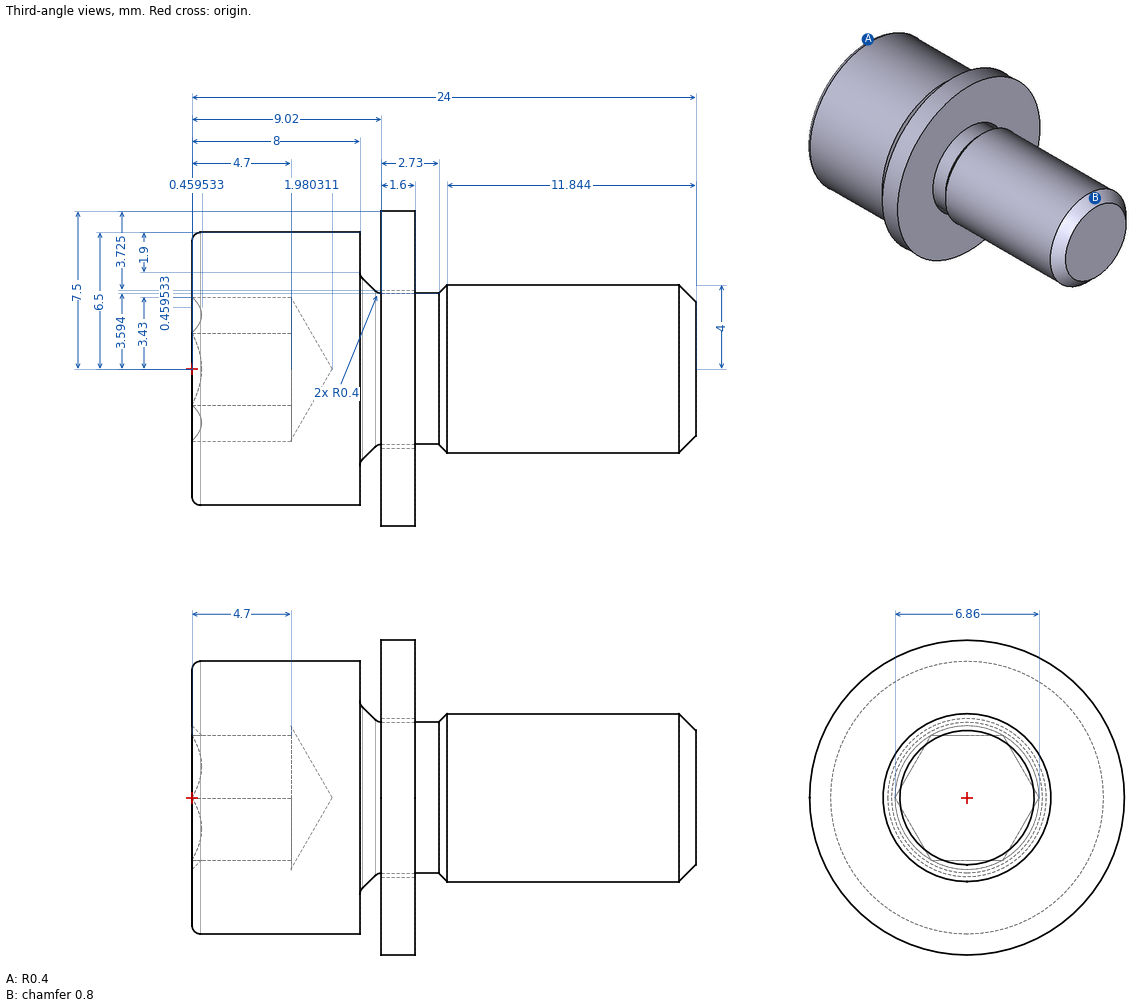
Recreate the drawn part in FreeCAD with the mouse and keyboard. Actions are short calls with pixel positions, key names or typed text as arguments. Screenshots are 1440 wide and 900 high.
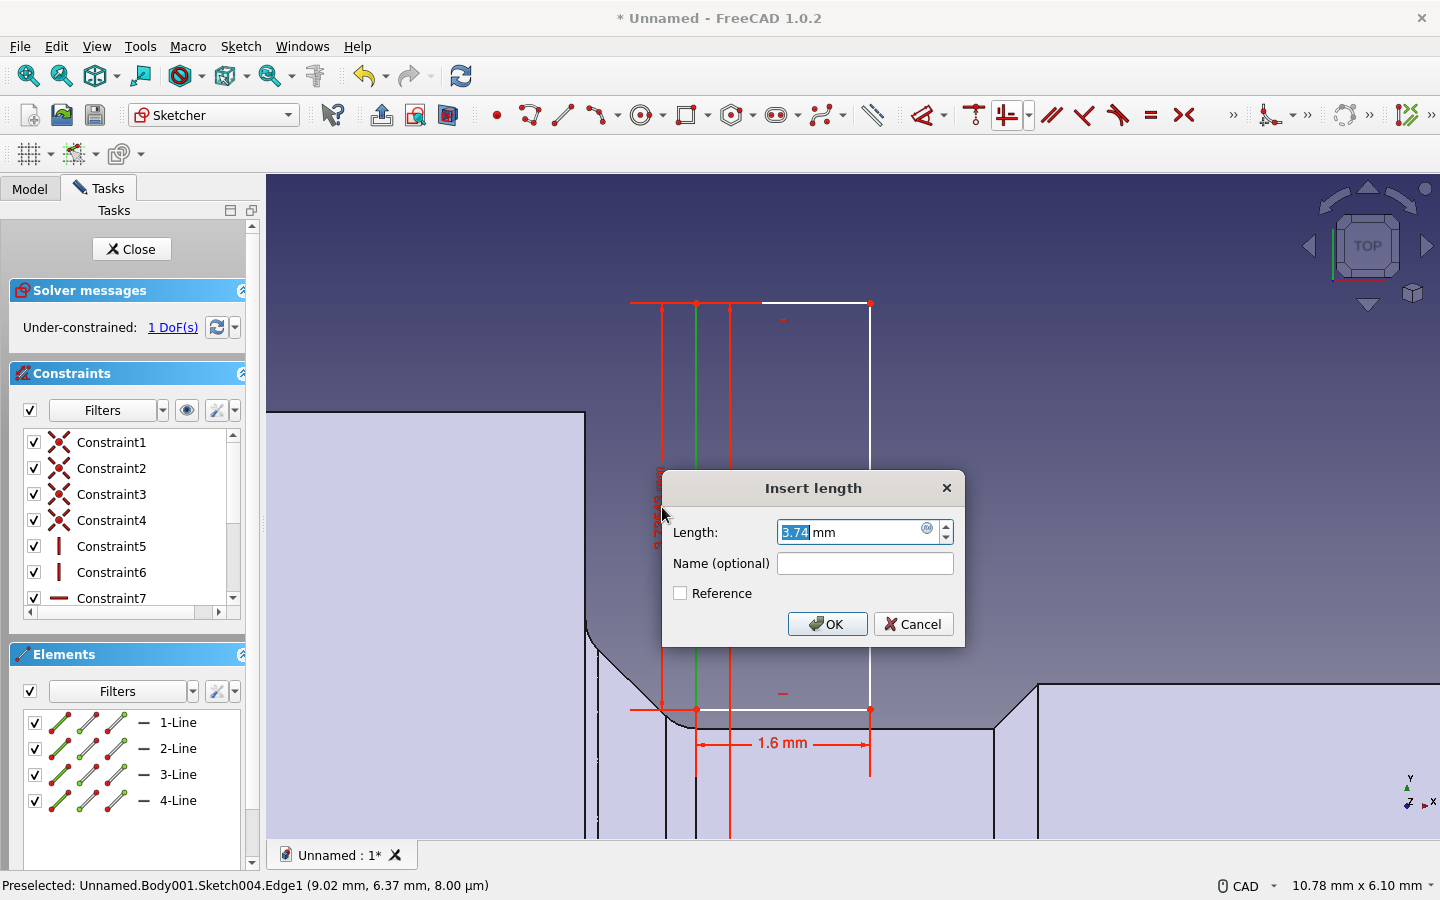
text(3.725)
key(Return)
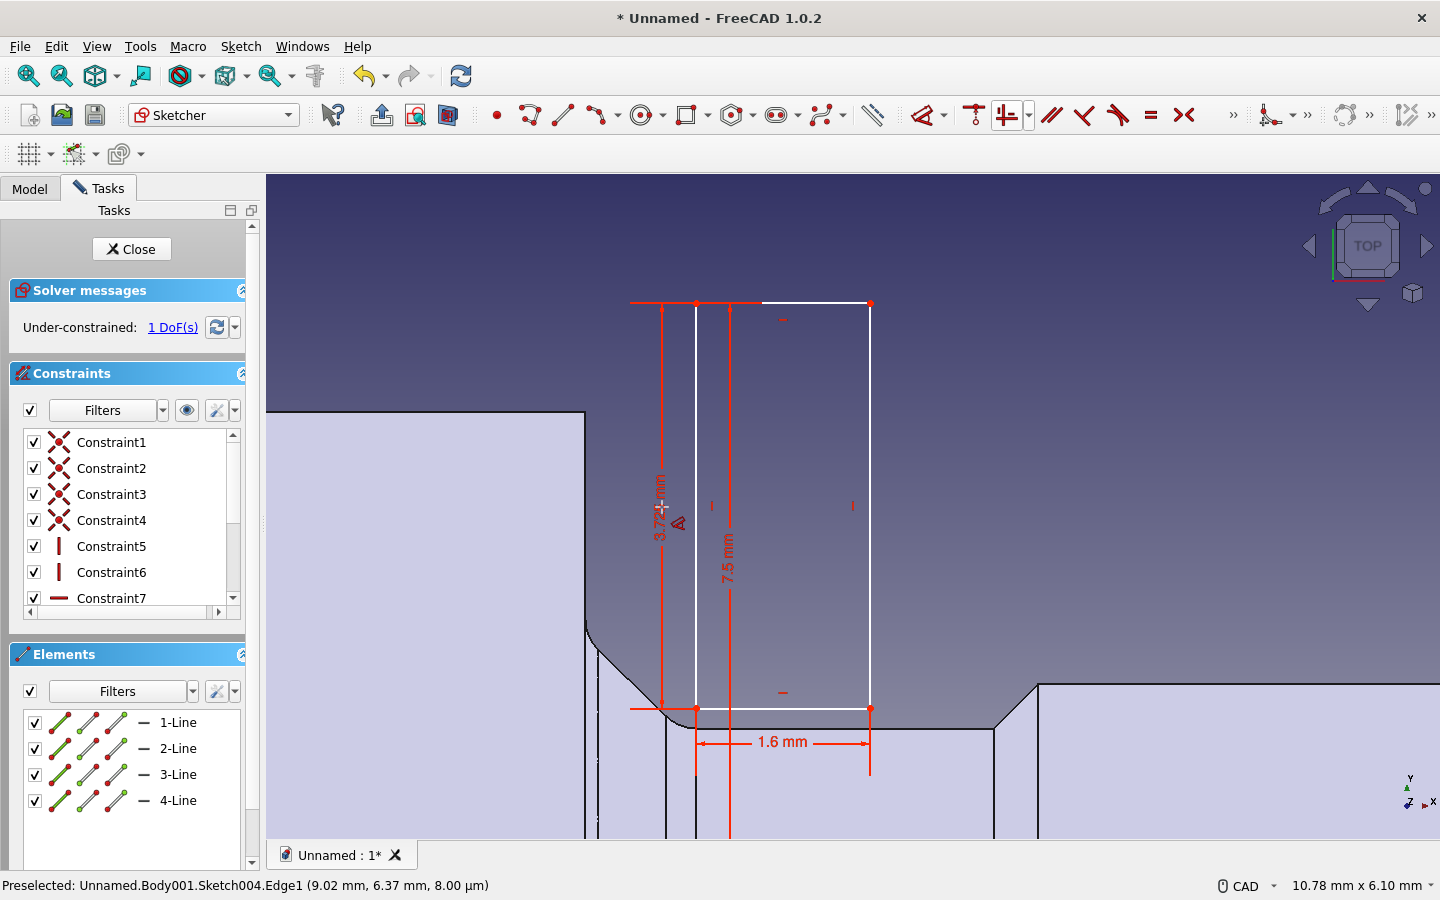
click(696, 303)
click(495, 269)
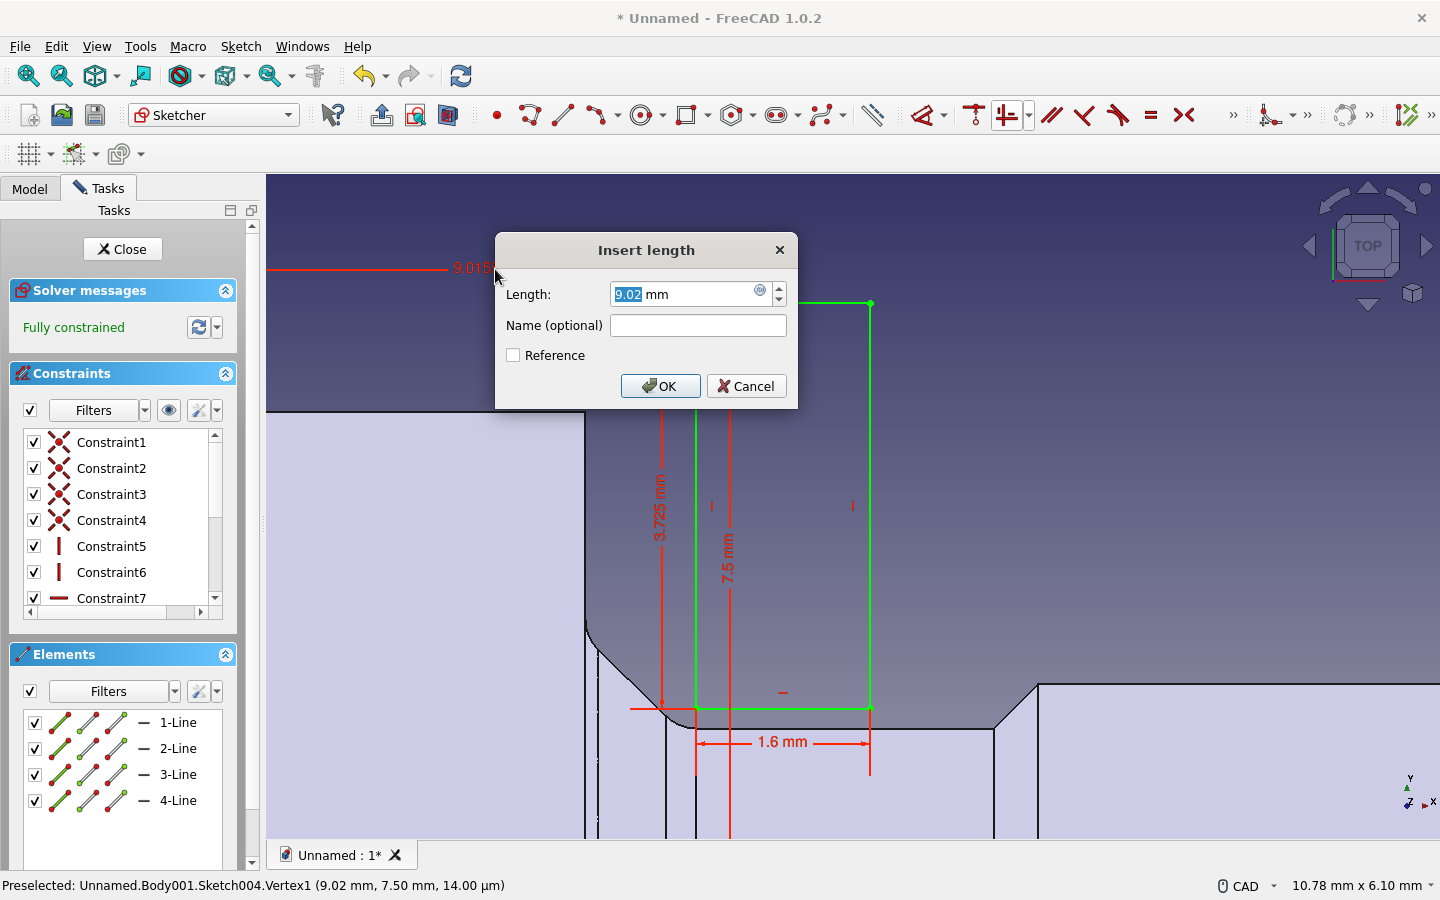
text(9.02)
key(Return)
key(Escape)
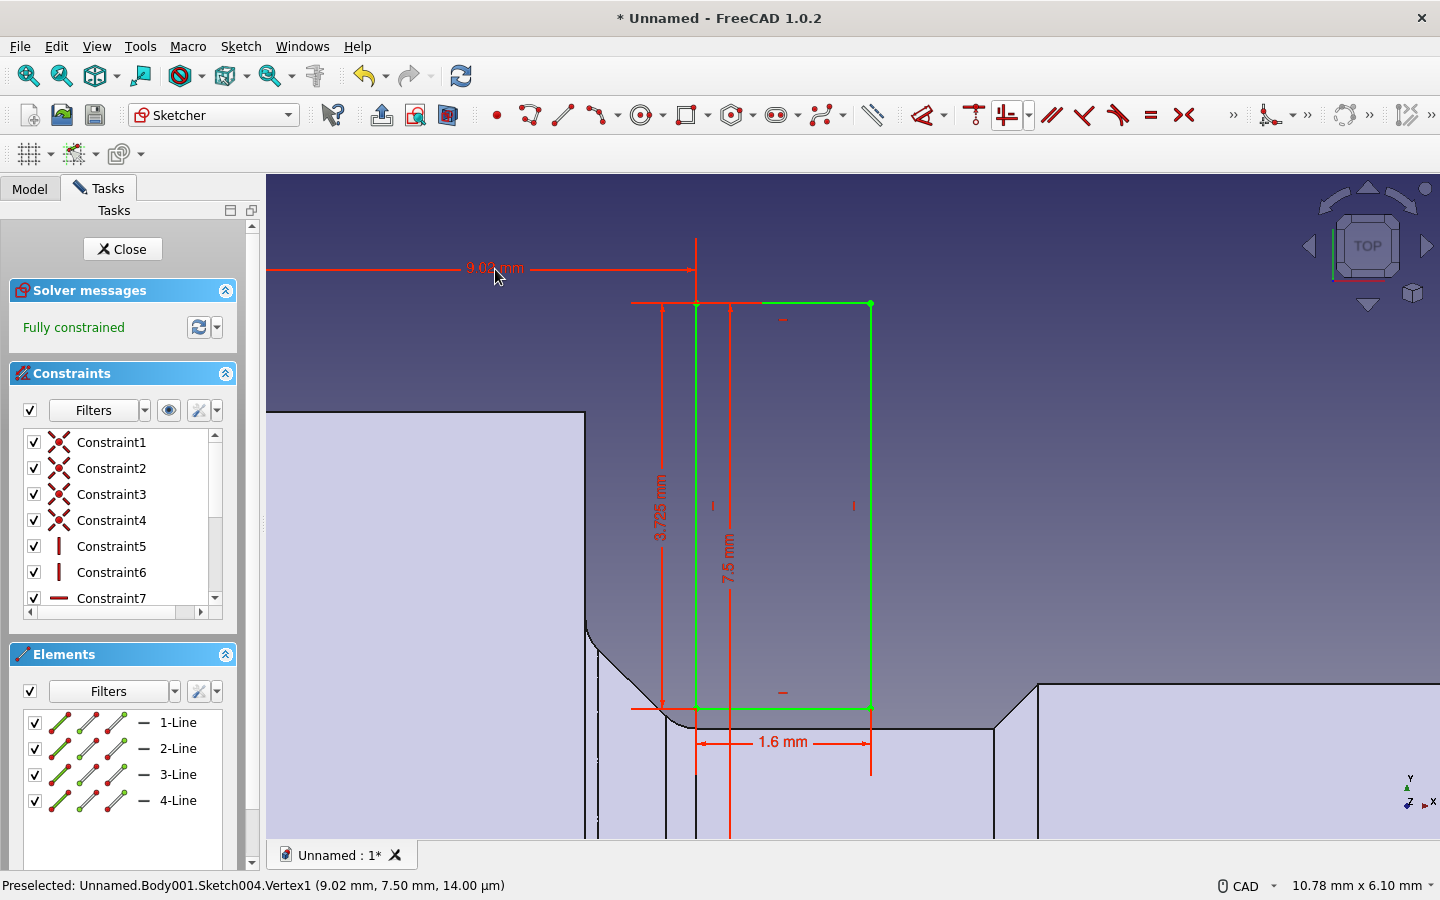
click(123, 249)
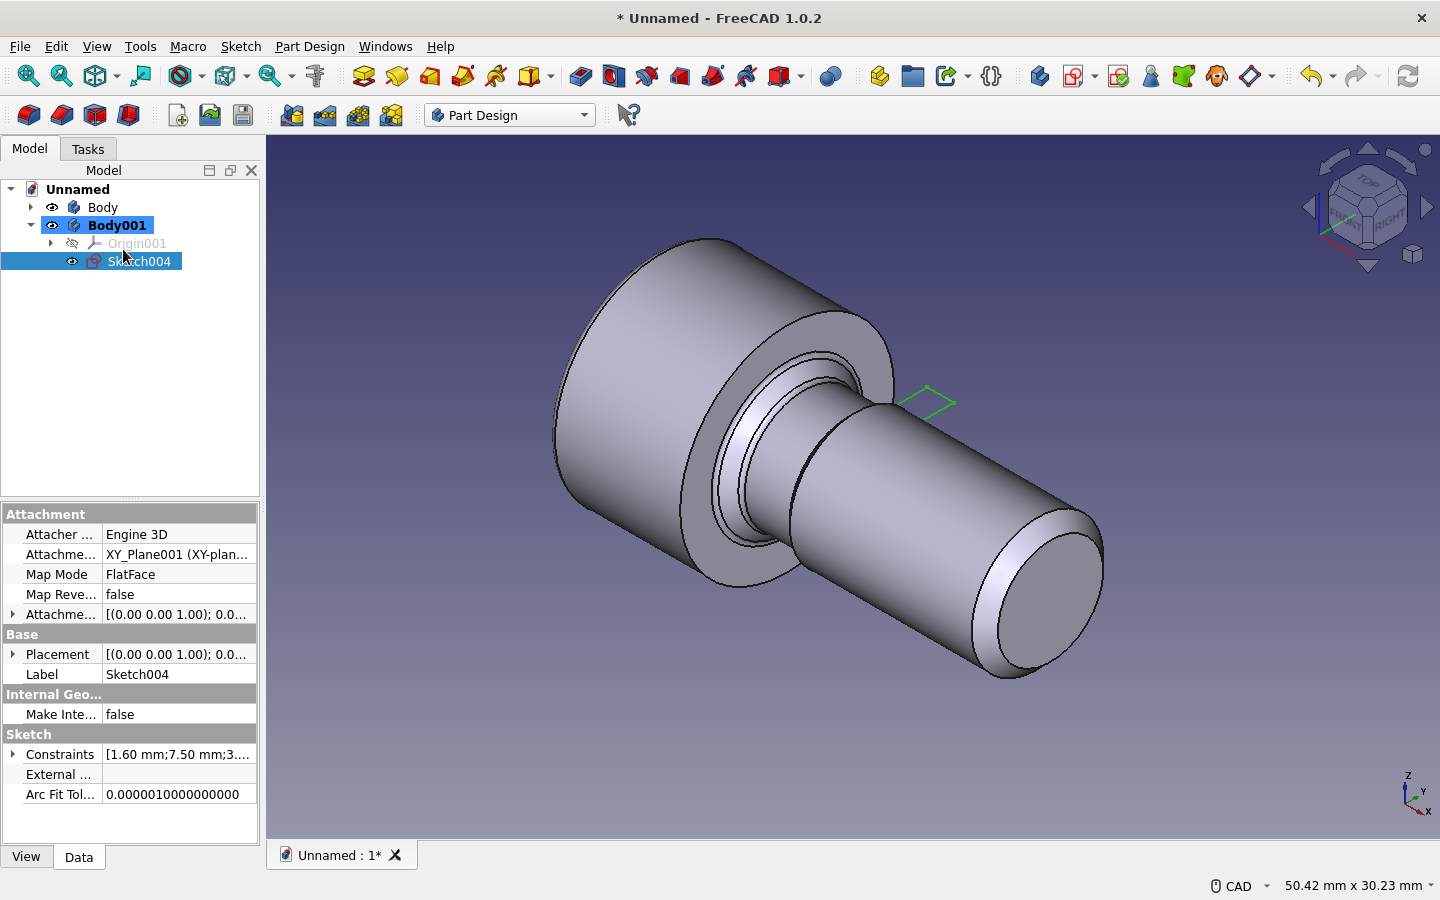
click(397, 76)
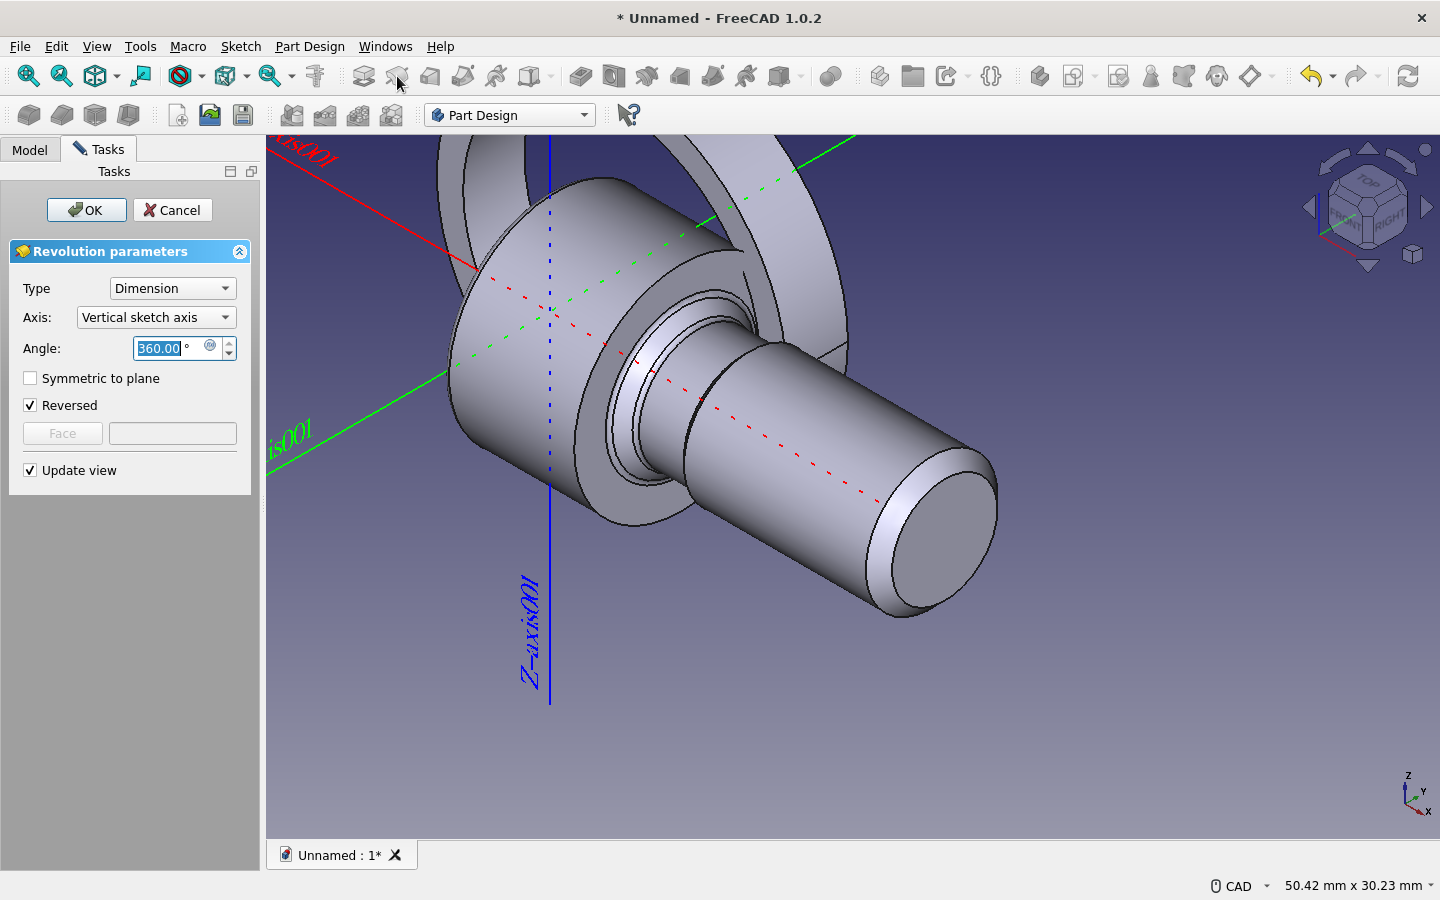
click(157, 318)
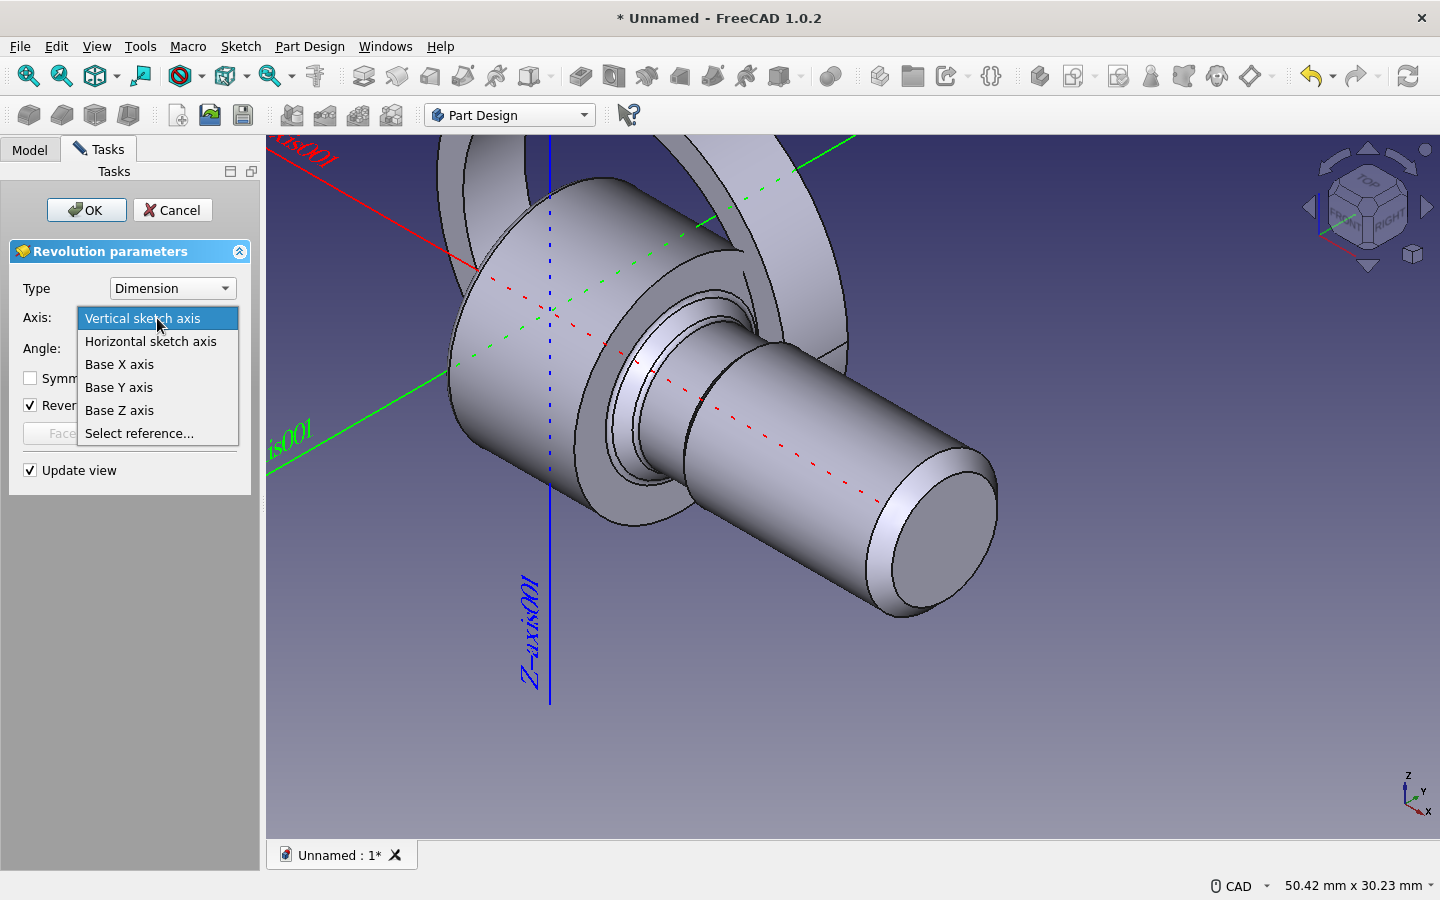
click(156, 342)